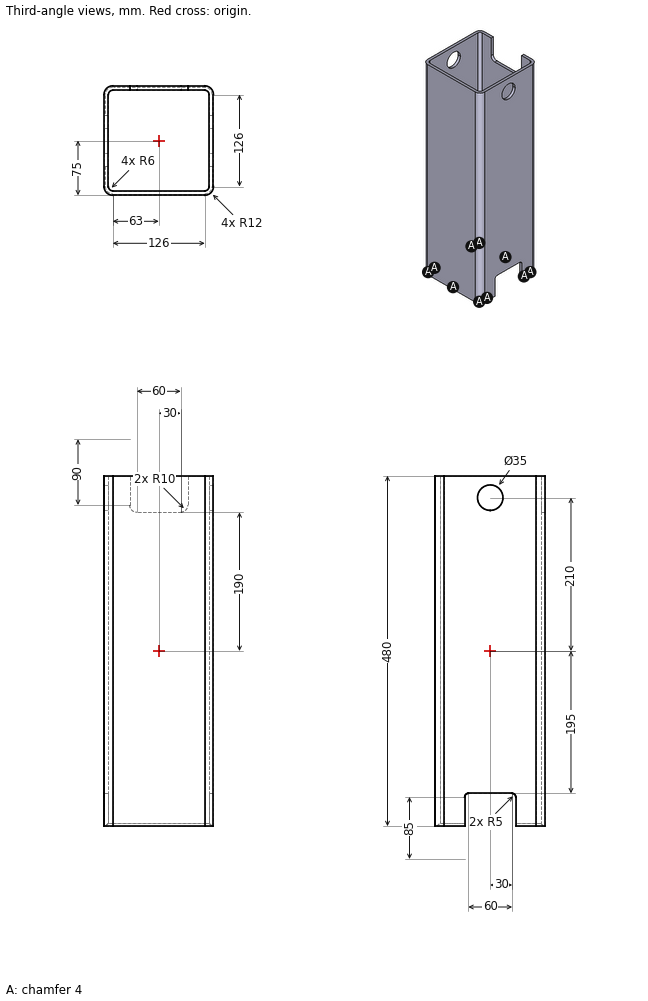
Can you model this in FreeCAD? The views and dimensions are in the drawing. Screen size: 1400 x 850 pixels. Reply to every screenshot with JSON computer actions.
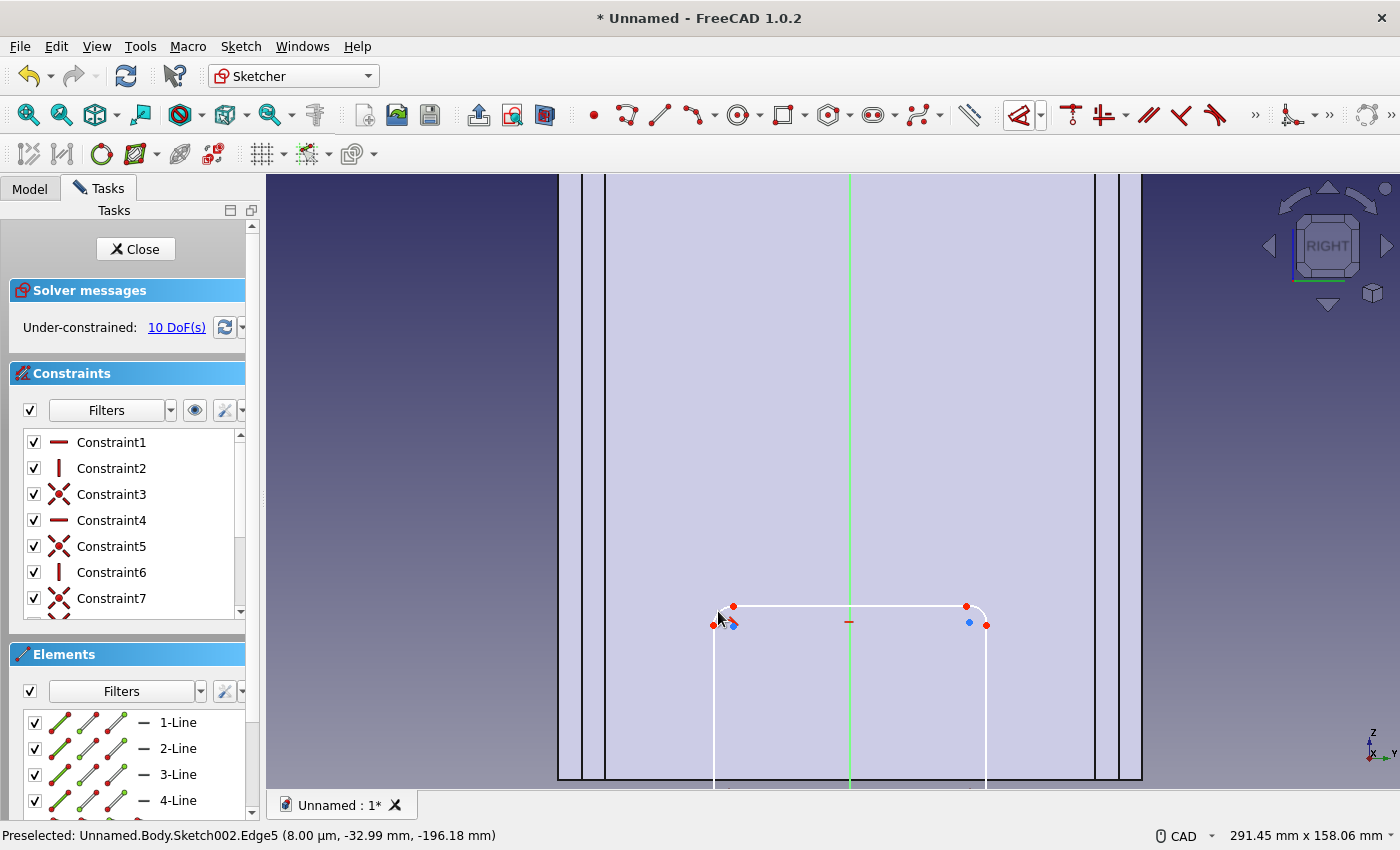
{"action": "scroll", "coordinate": [743, 614], "scroll_direction": "down", "scroll_amount": 8}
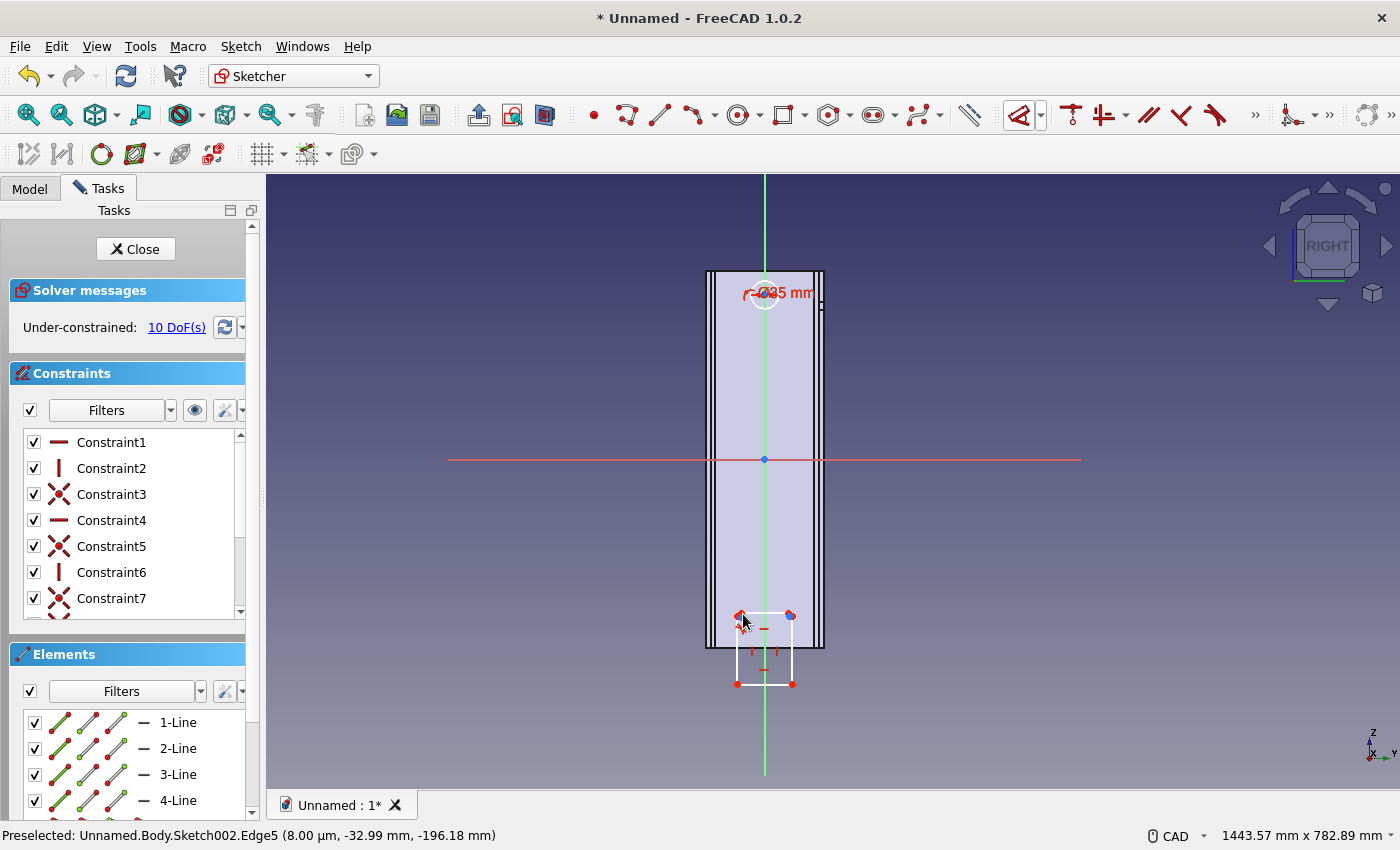
{"action": "scroll", "coordinate": [774, 613], "scroll_direction": "up", "scroll_amount": 2}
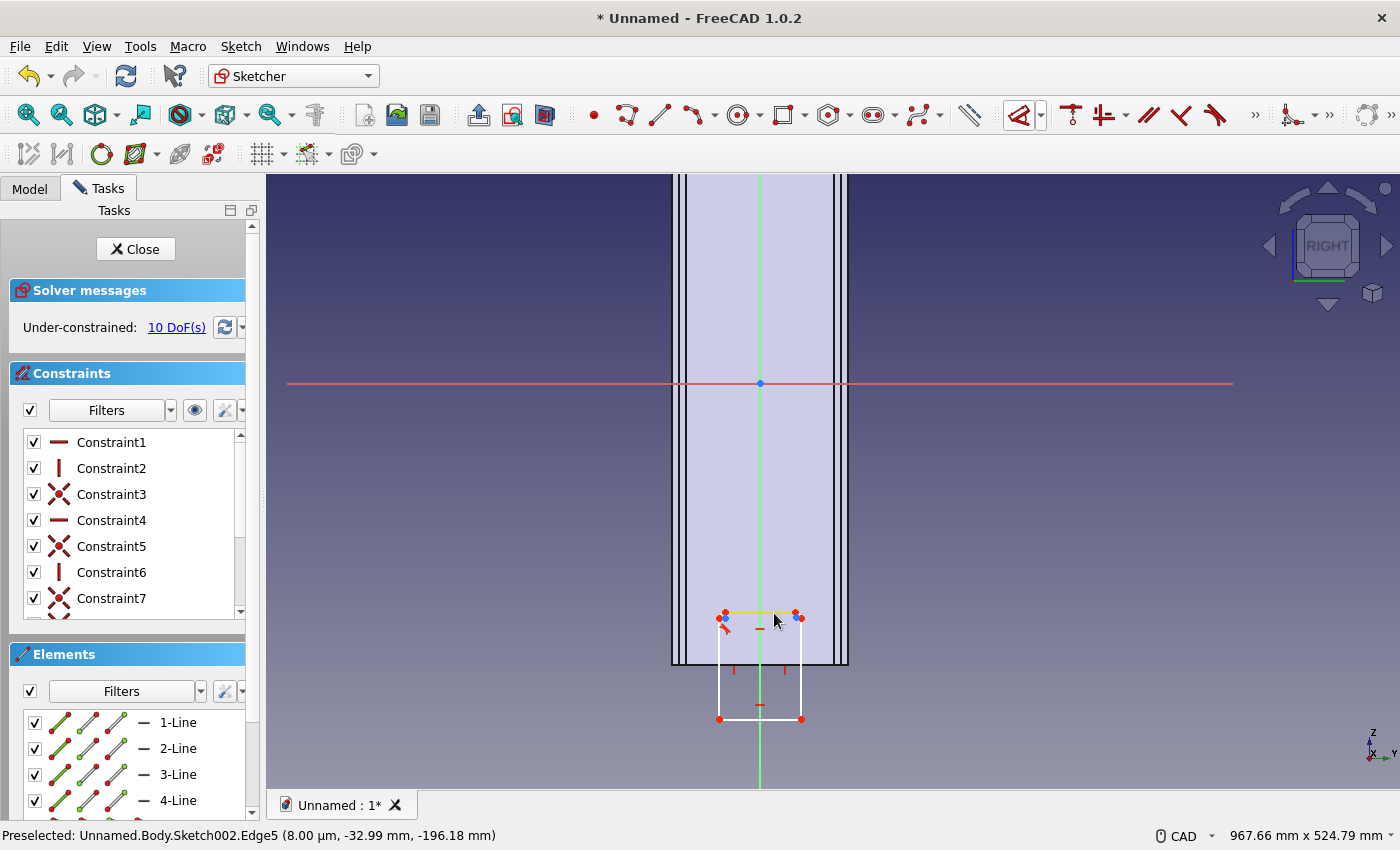
{"action": "left_click", "coordinate": [774, 613]}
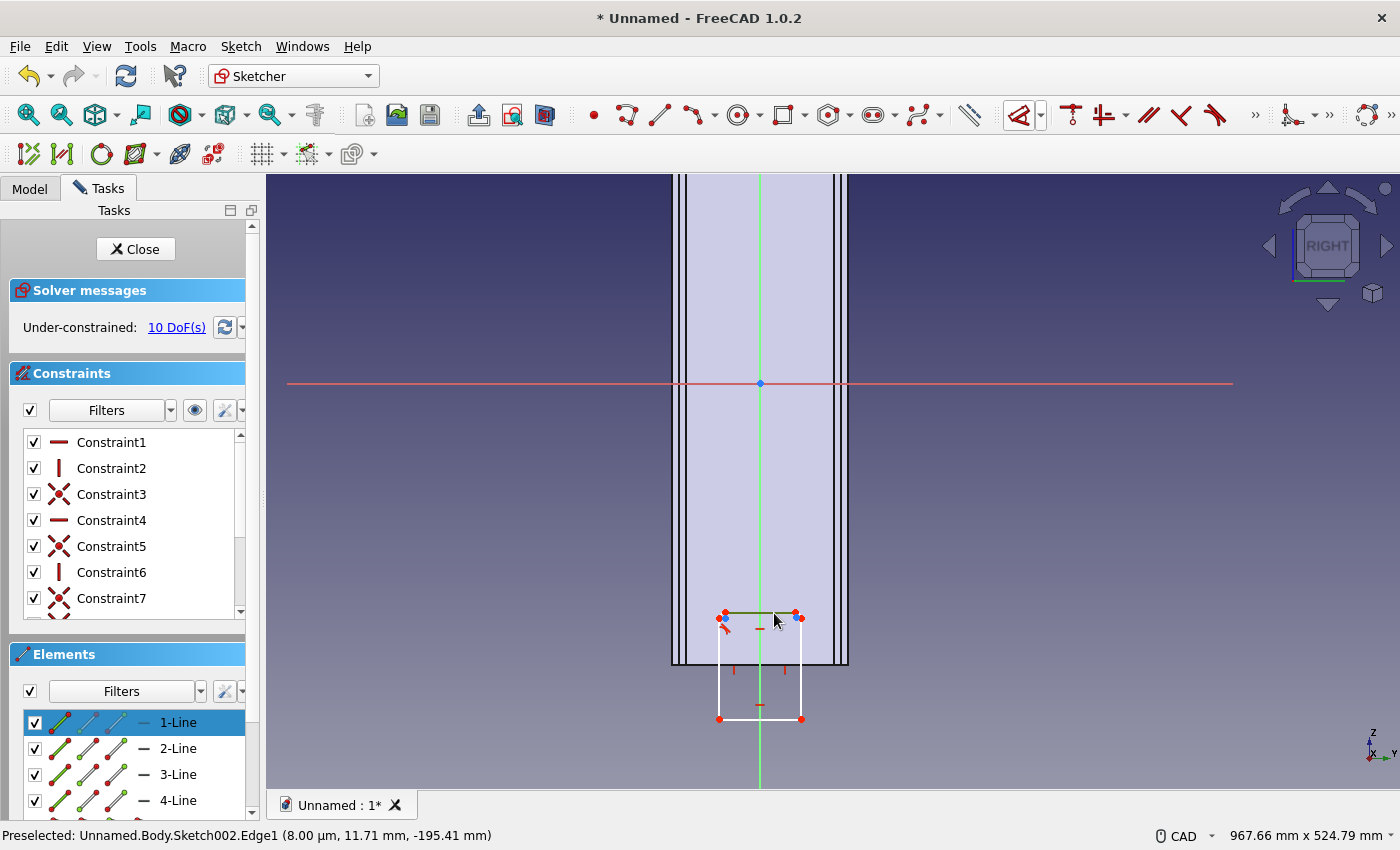
{"action": "scroll", "coordinate": [800, 614], "scroll_direction": "up", "scroll_amount": 6}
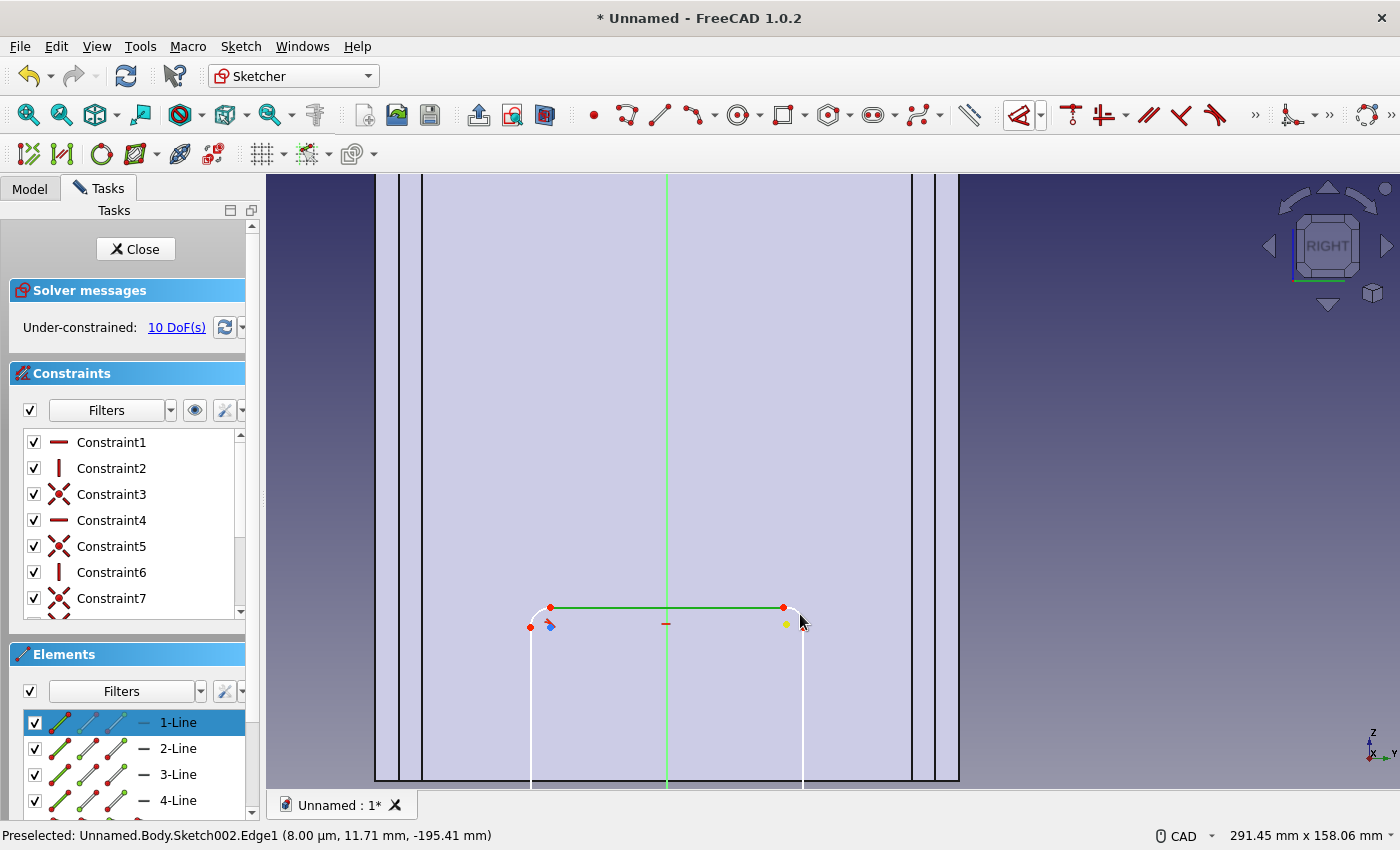
{"action": "left_click", "coordinate": [798, 612]}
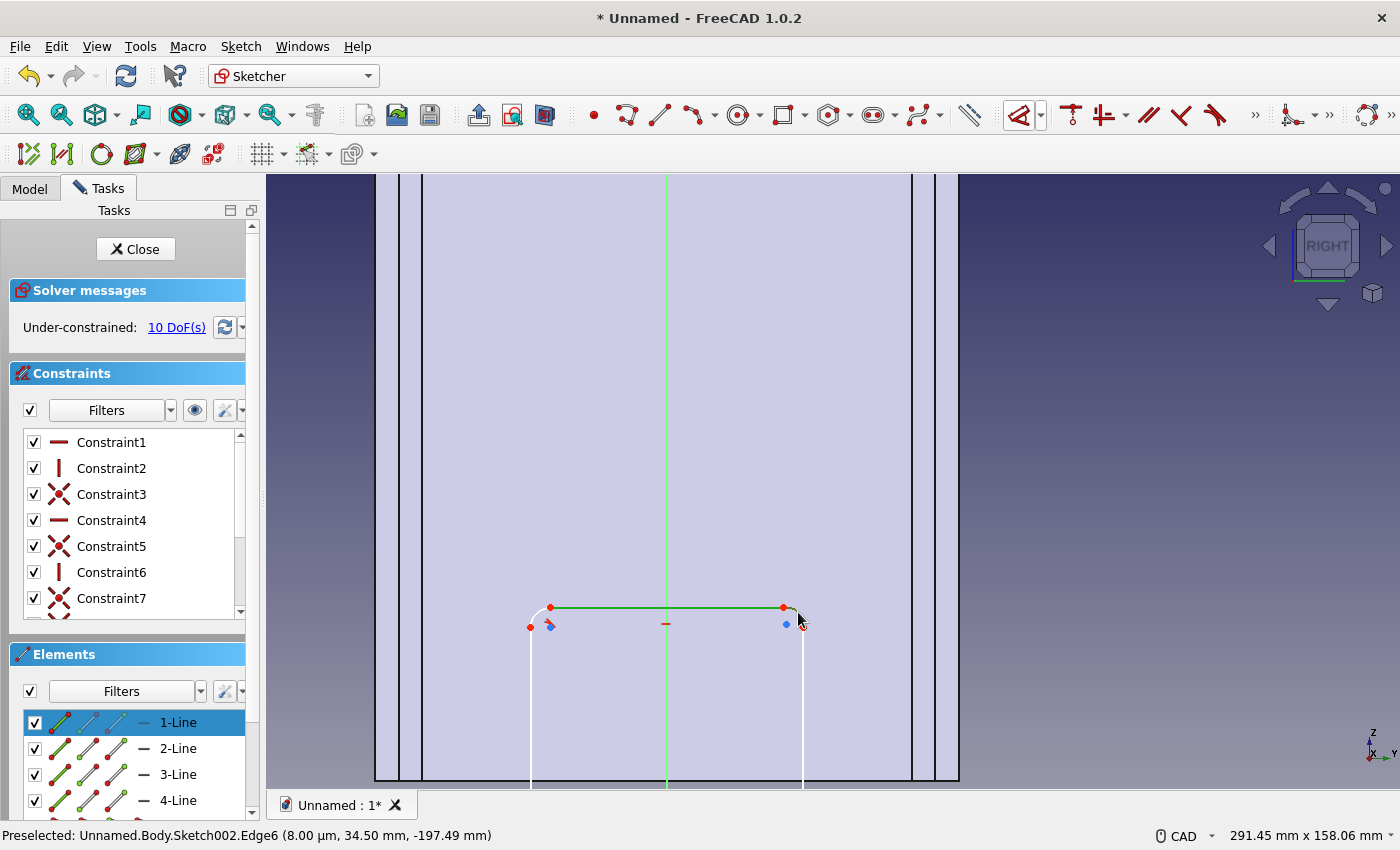
{"action": "key", "text": "t"}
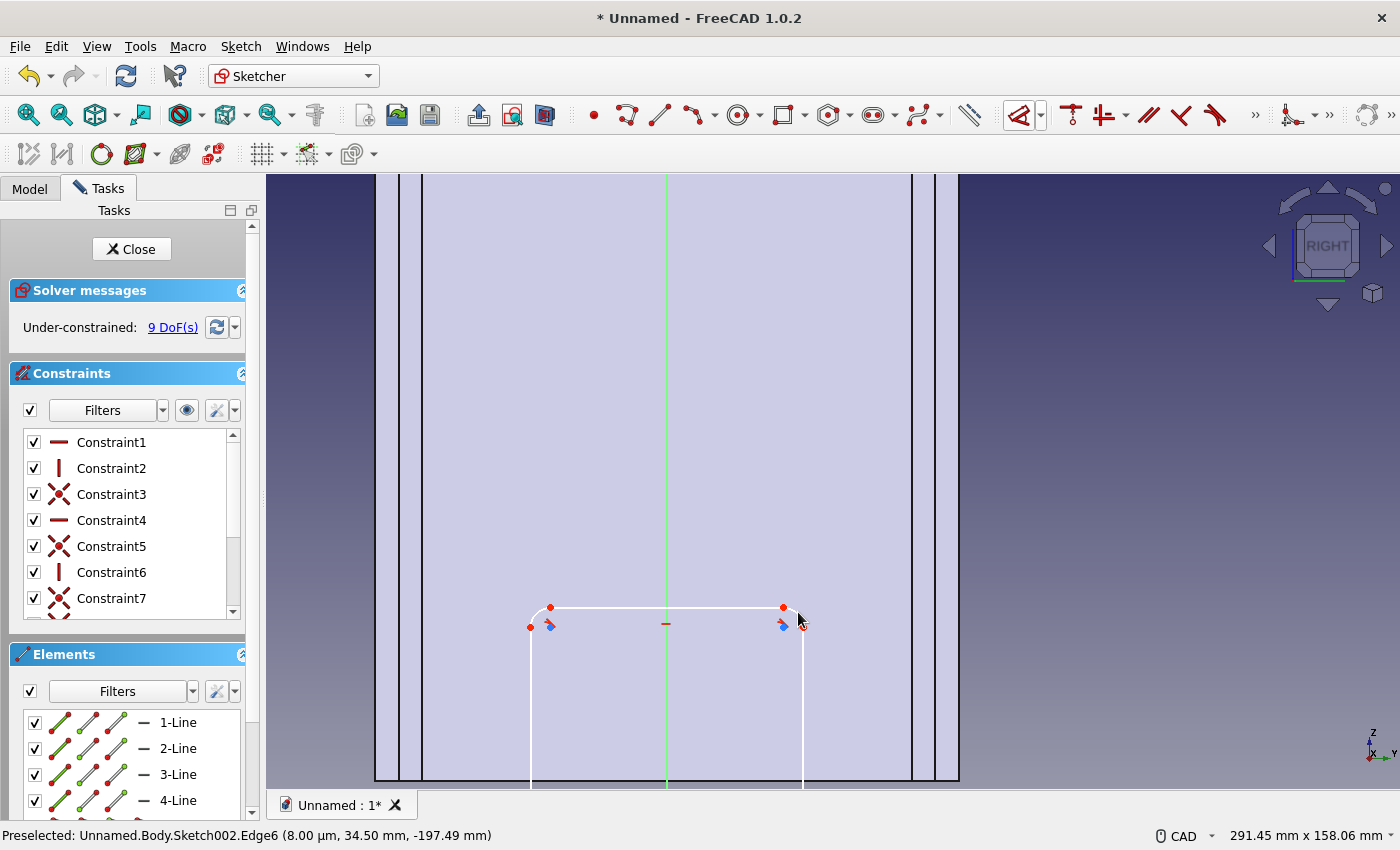
{"action": "scroll", "coordinate": [789, 614], "scroll_direction": "down", "scroll_amount": 8}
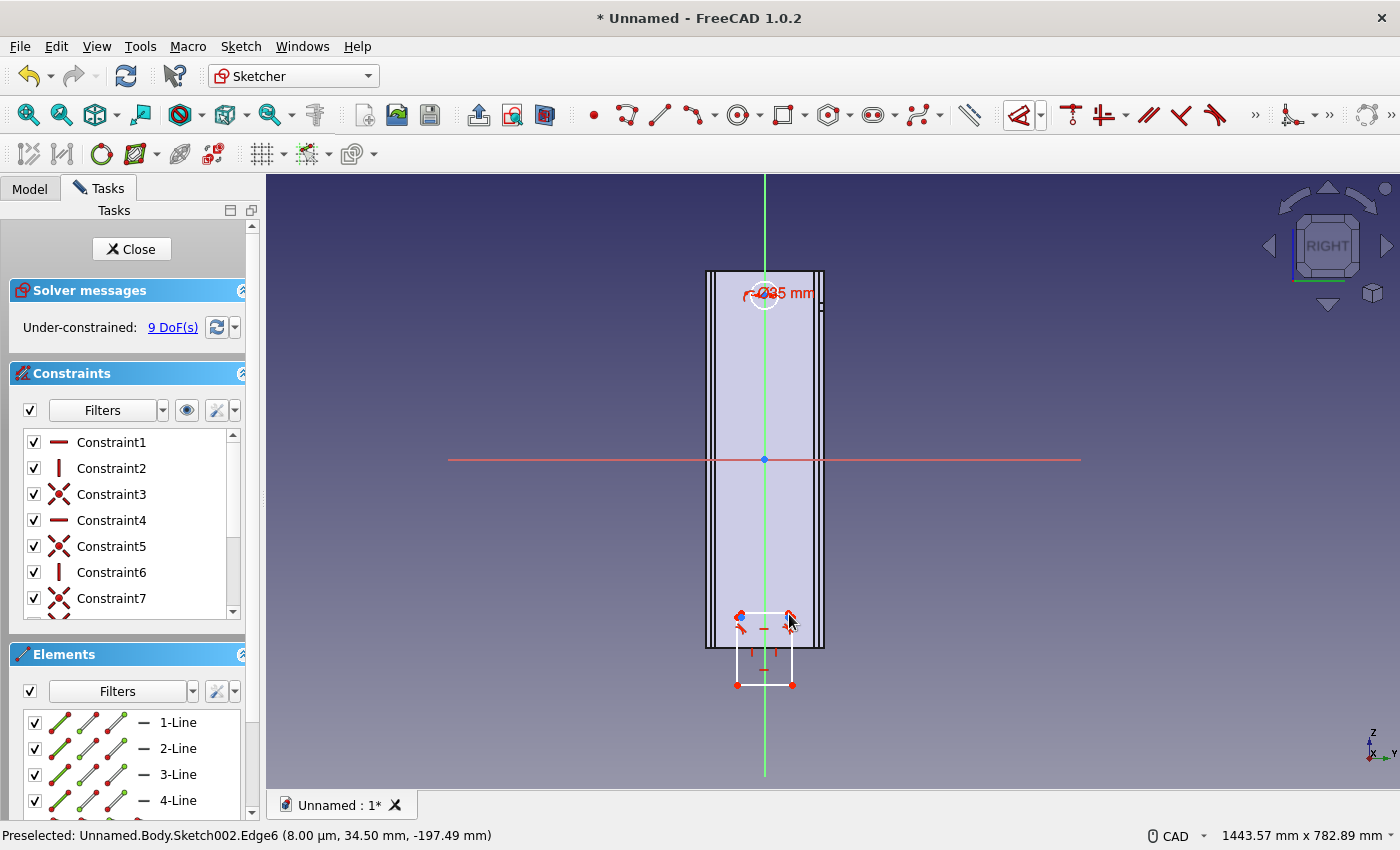
{"action": "left_click", "coordinate": [737, 638]}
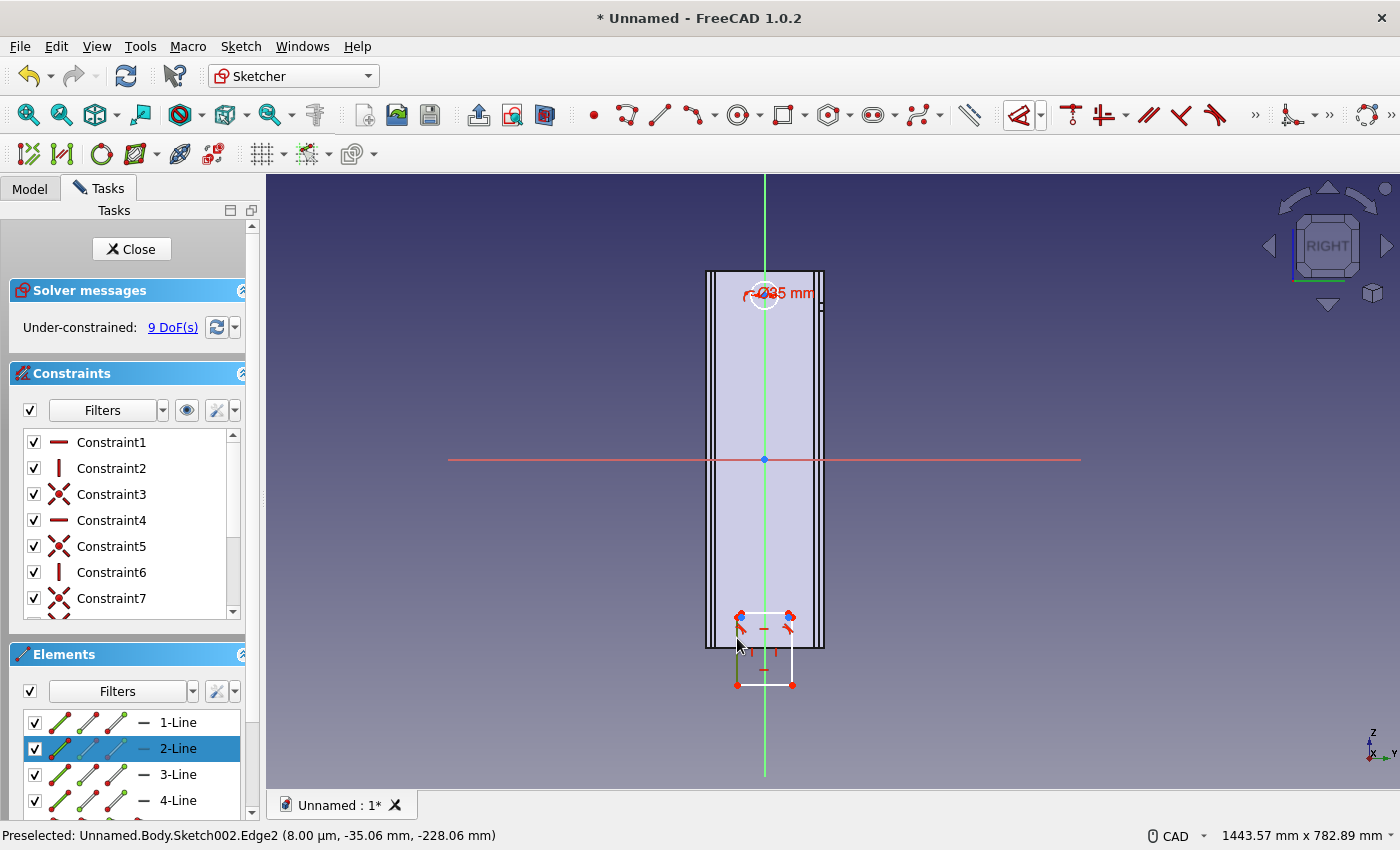
{"action": "scroll", "coordinate": [738, 615], "scroll_direction": "up", "scroll_amount": 8}